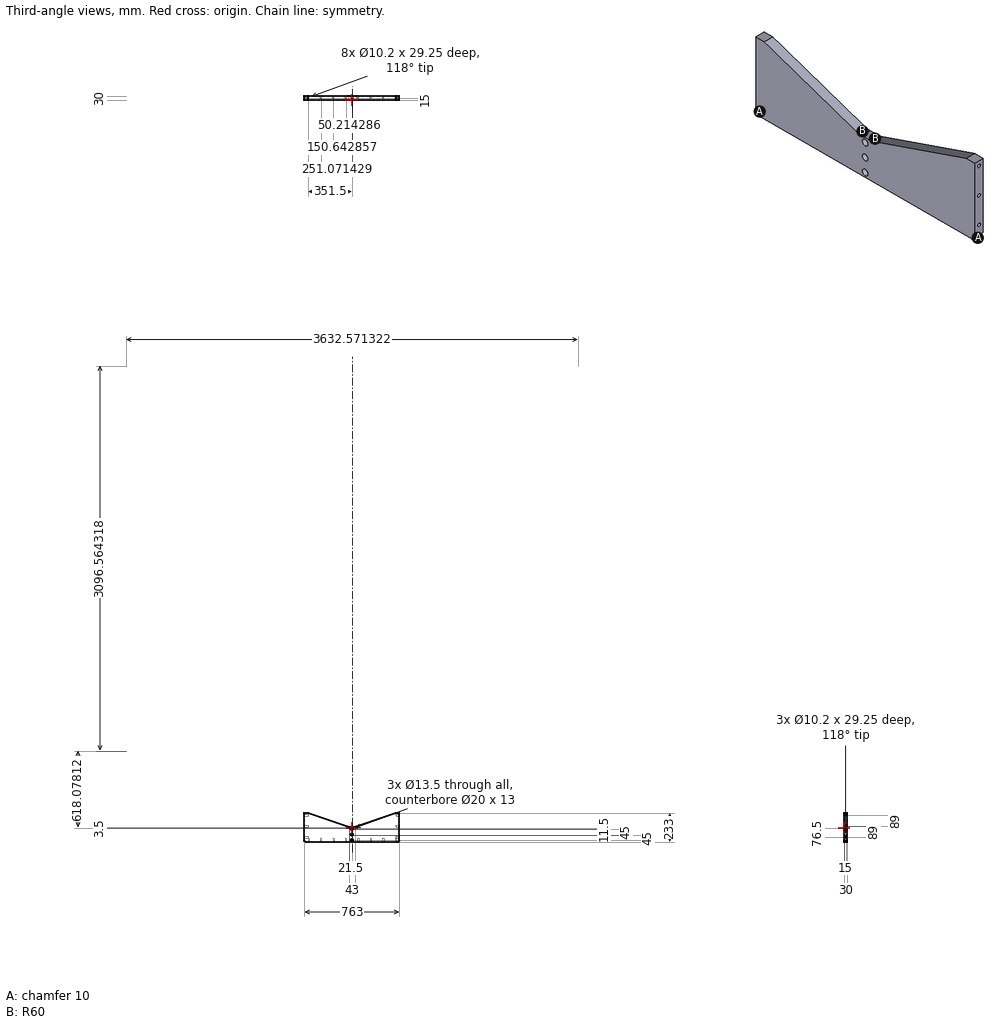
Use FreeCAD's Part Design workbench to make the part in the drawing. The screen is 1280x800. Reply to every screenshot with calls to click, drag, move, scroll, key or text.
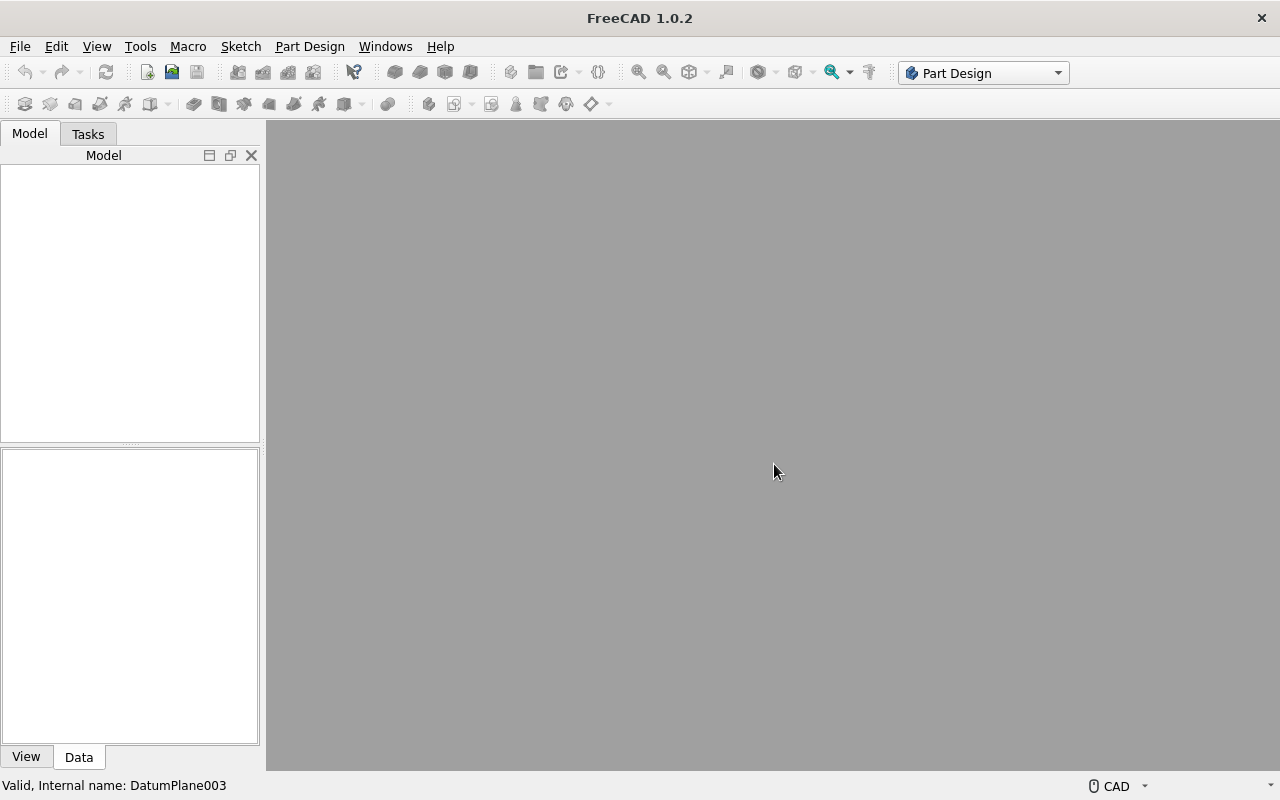
key(ctrl+n)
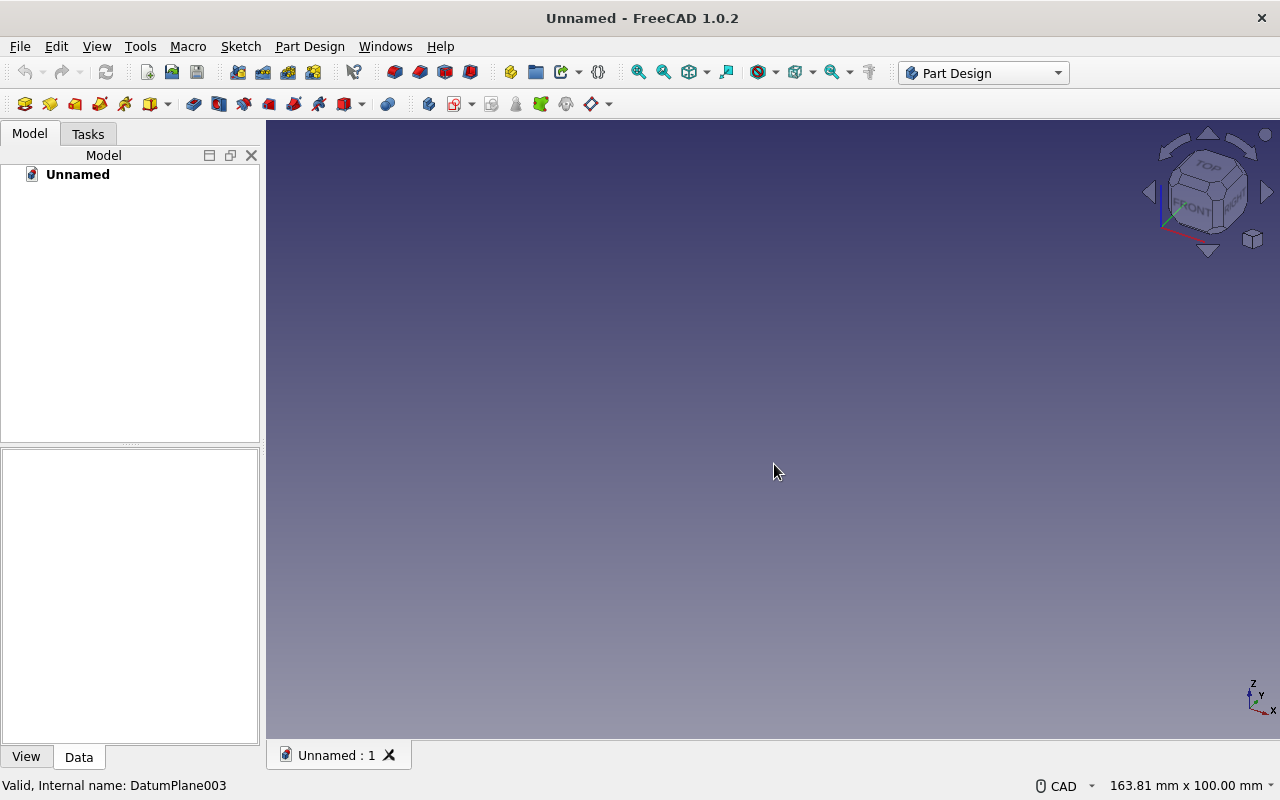
click(454, 104)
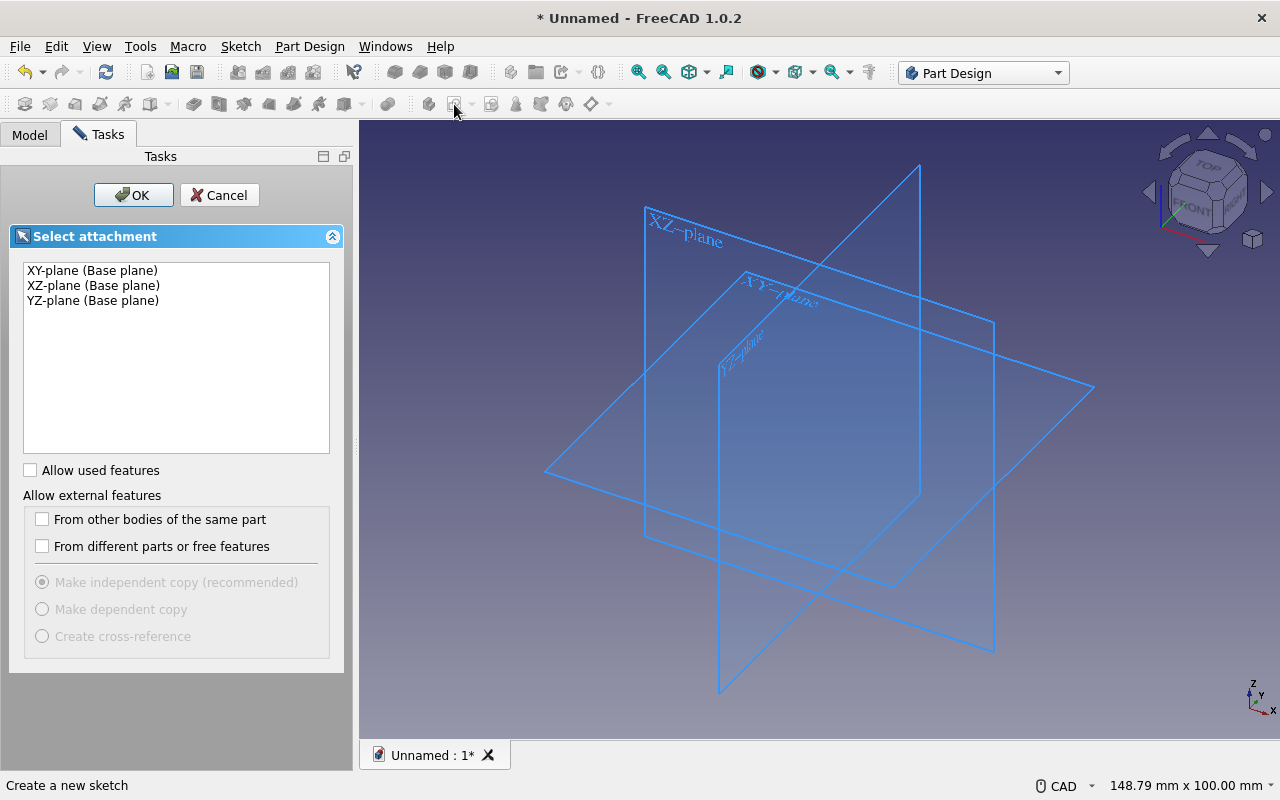
click(84, 286)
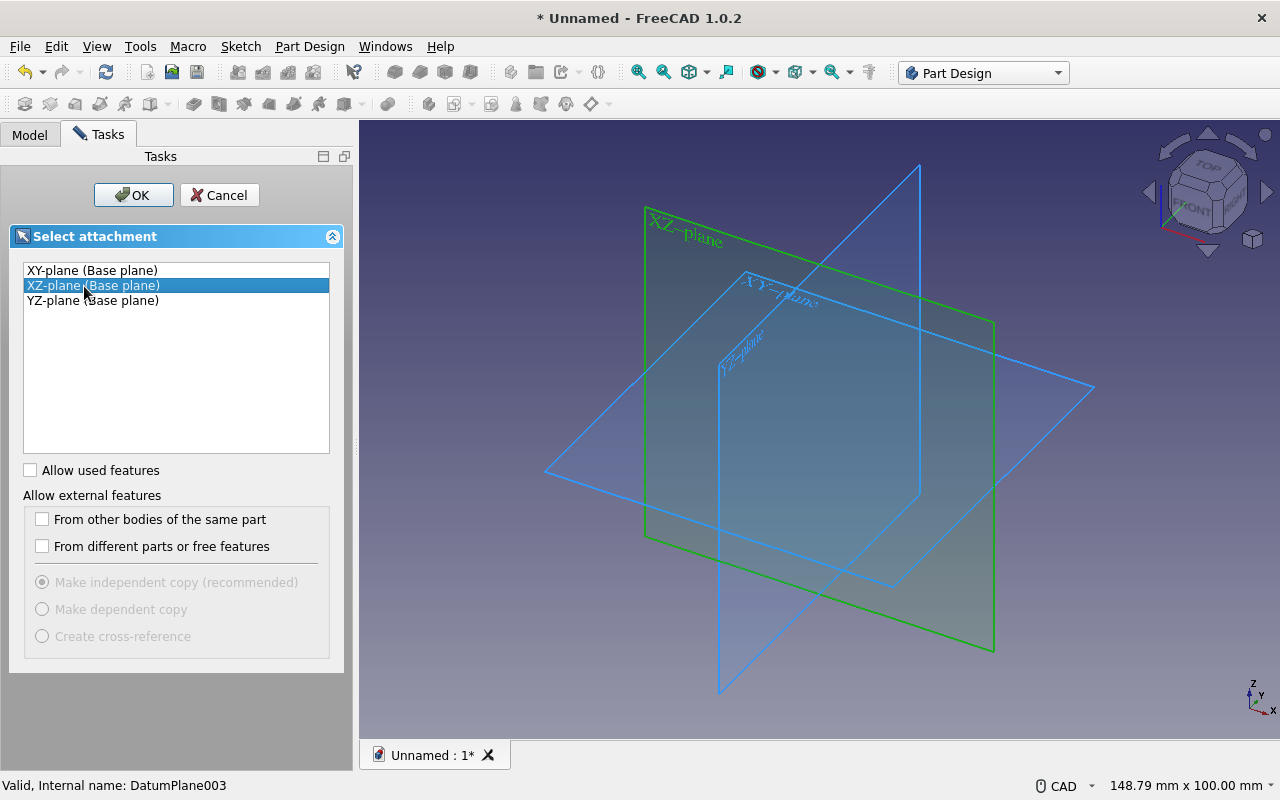
click(134, 195)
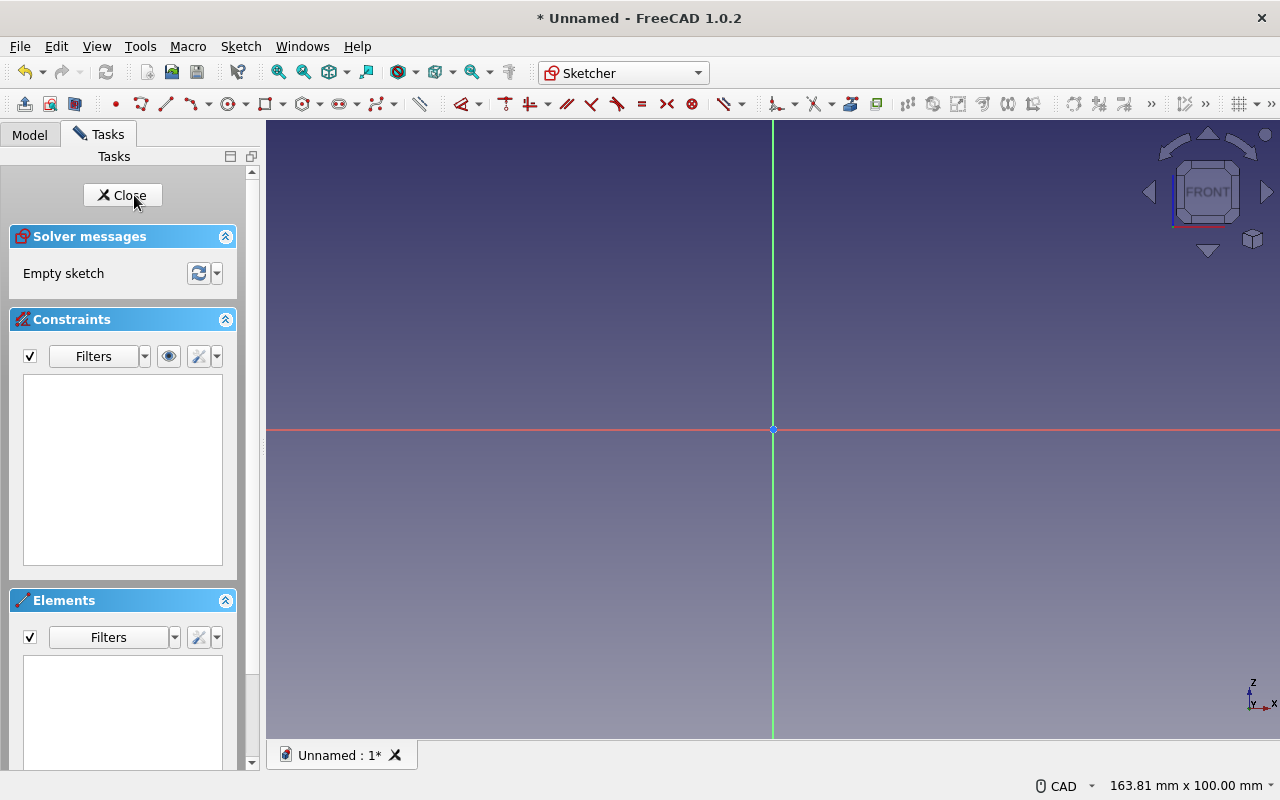
scroll(694, 430, down, 10)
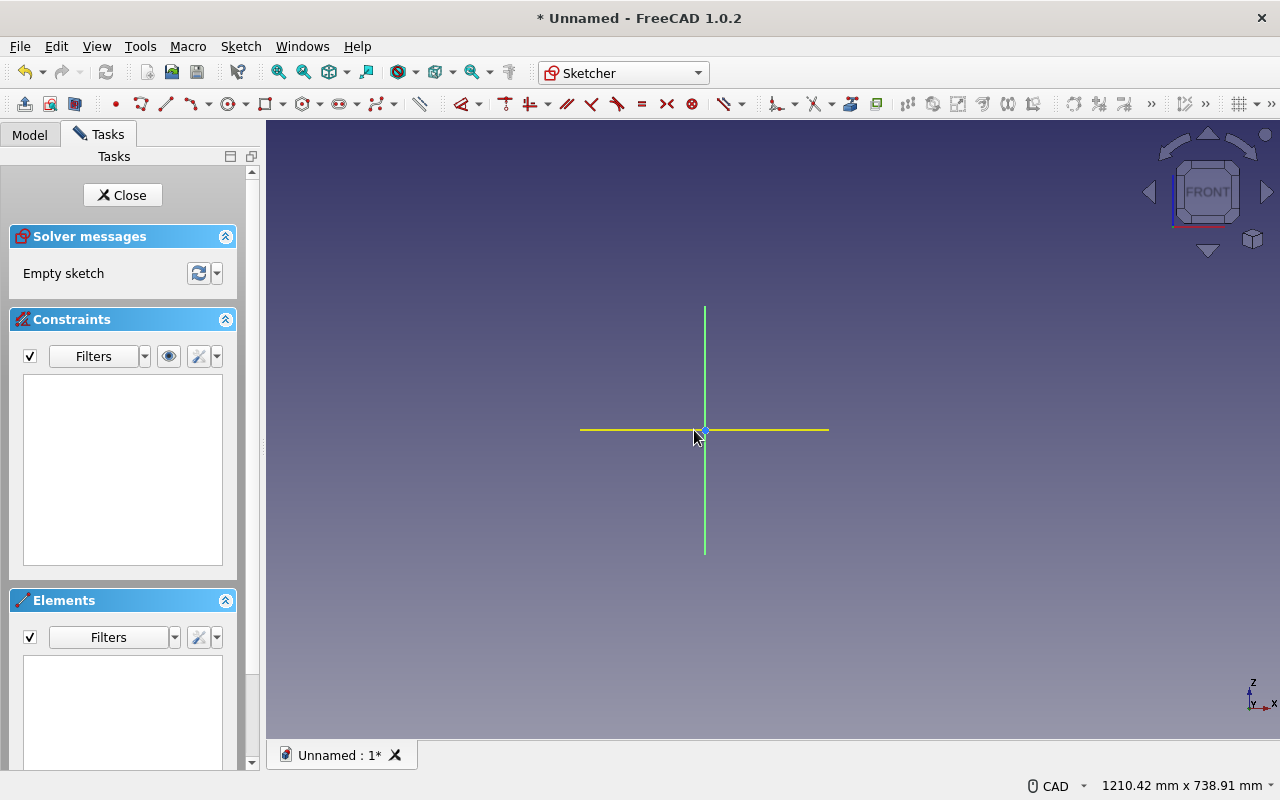
key(g)
key(v)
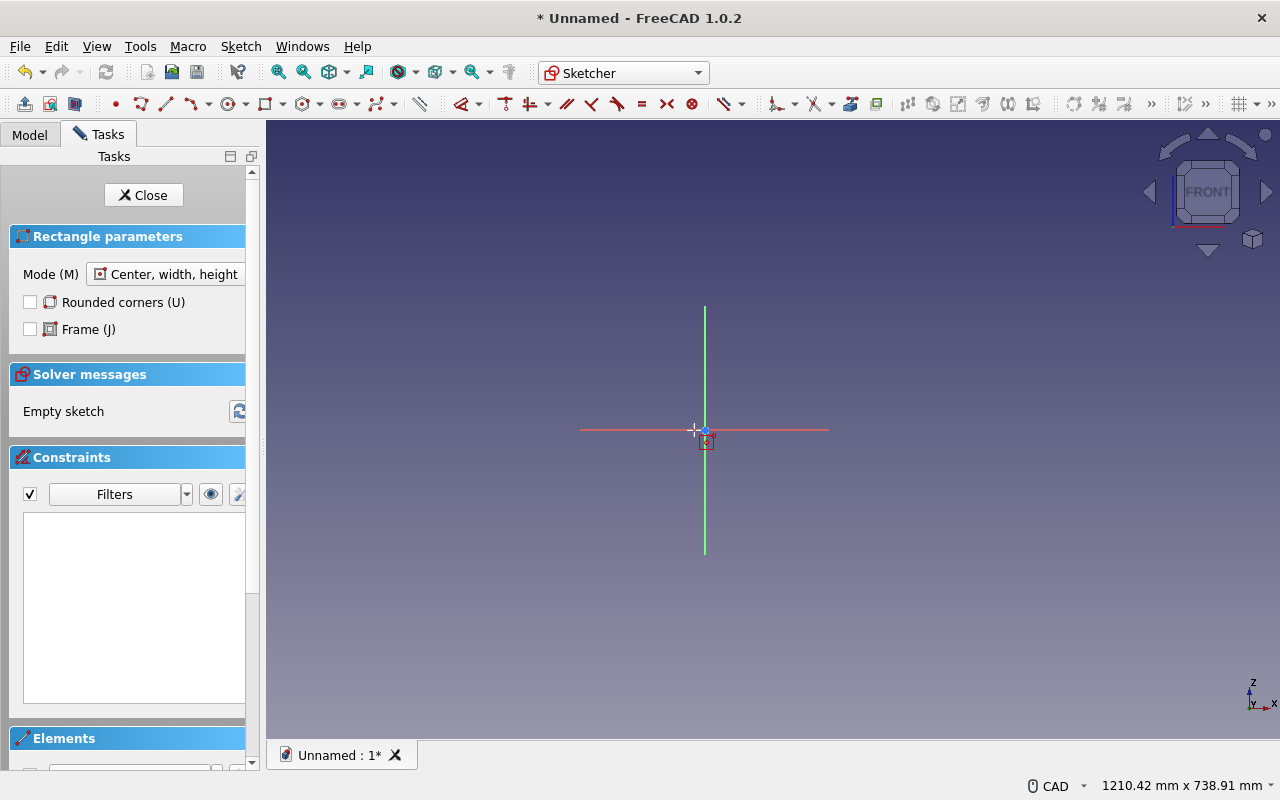
click(705, 430)
click(1025, 333)
key(Escape)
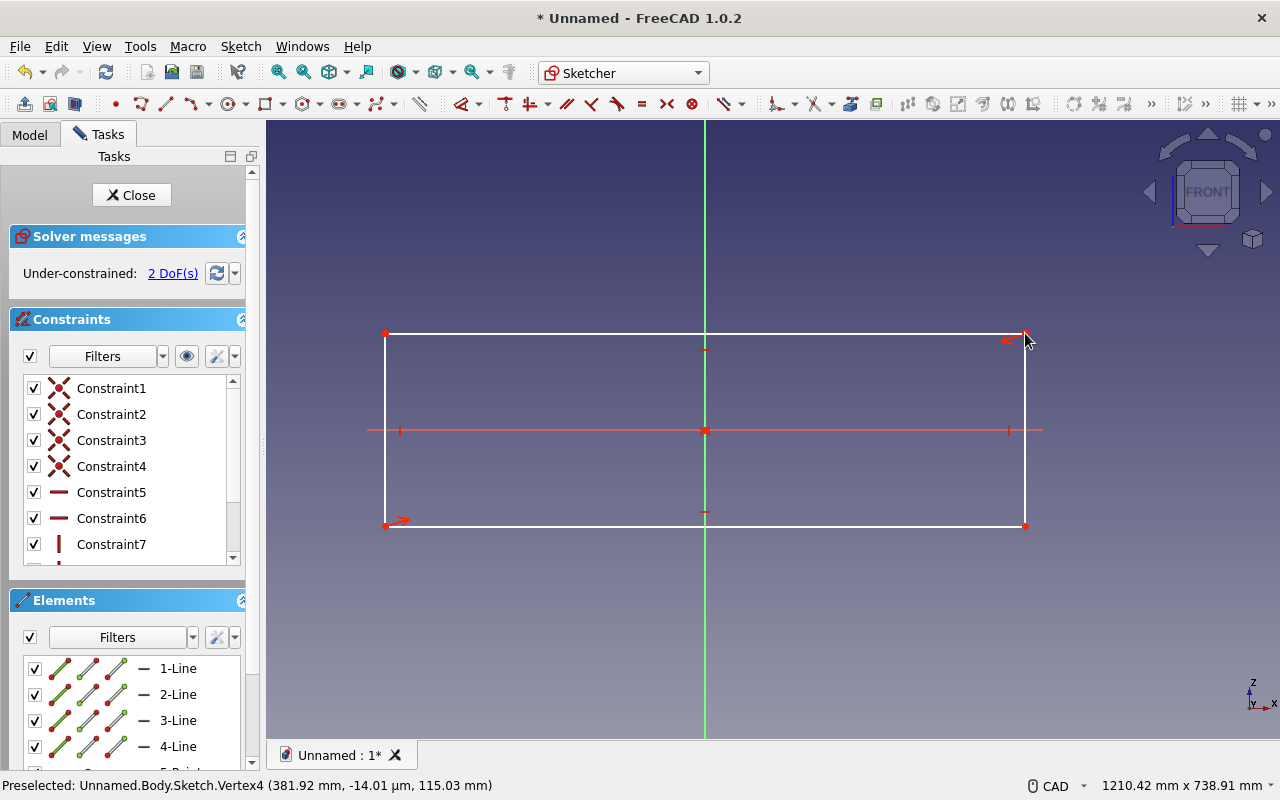
key(d)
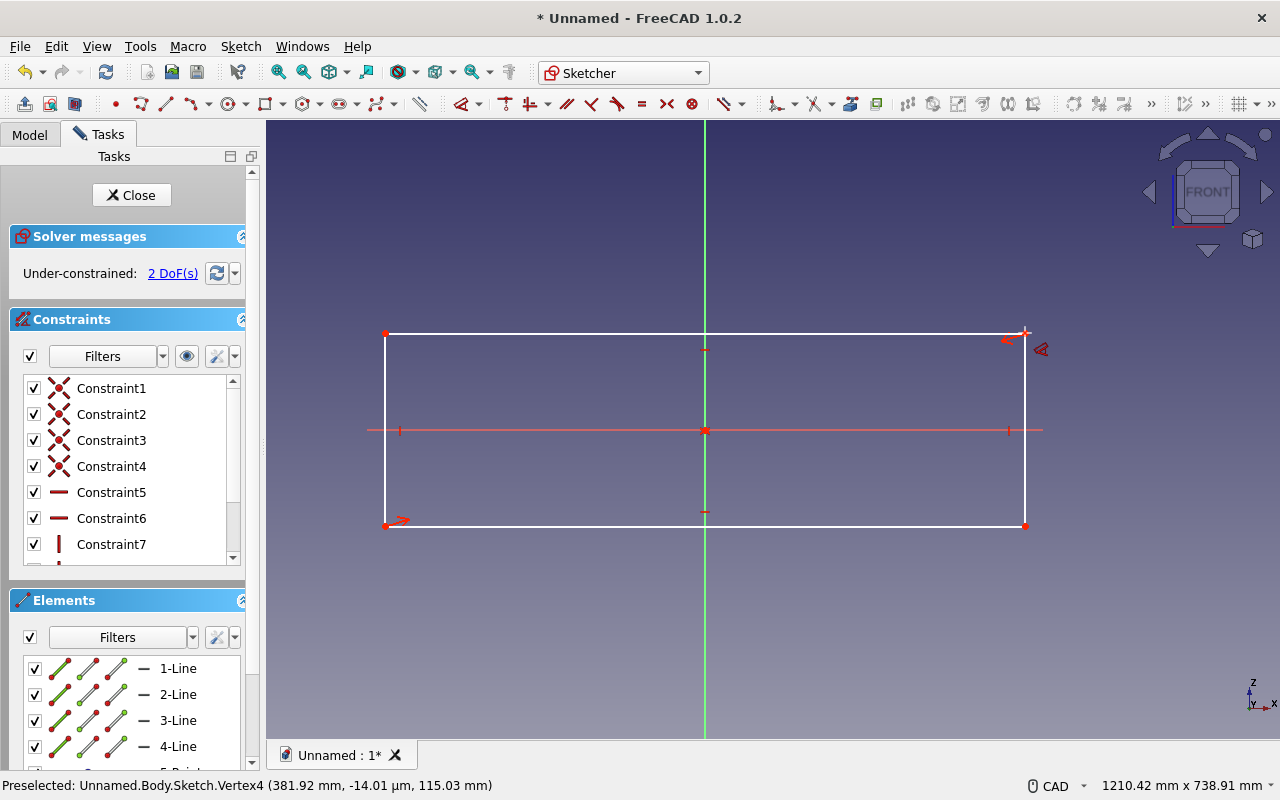
click(577, 527)
click(558, 561)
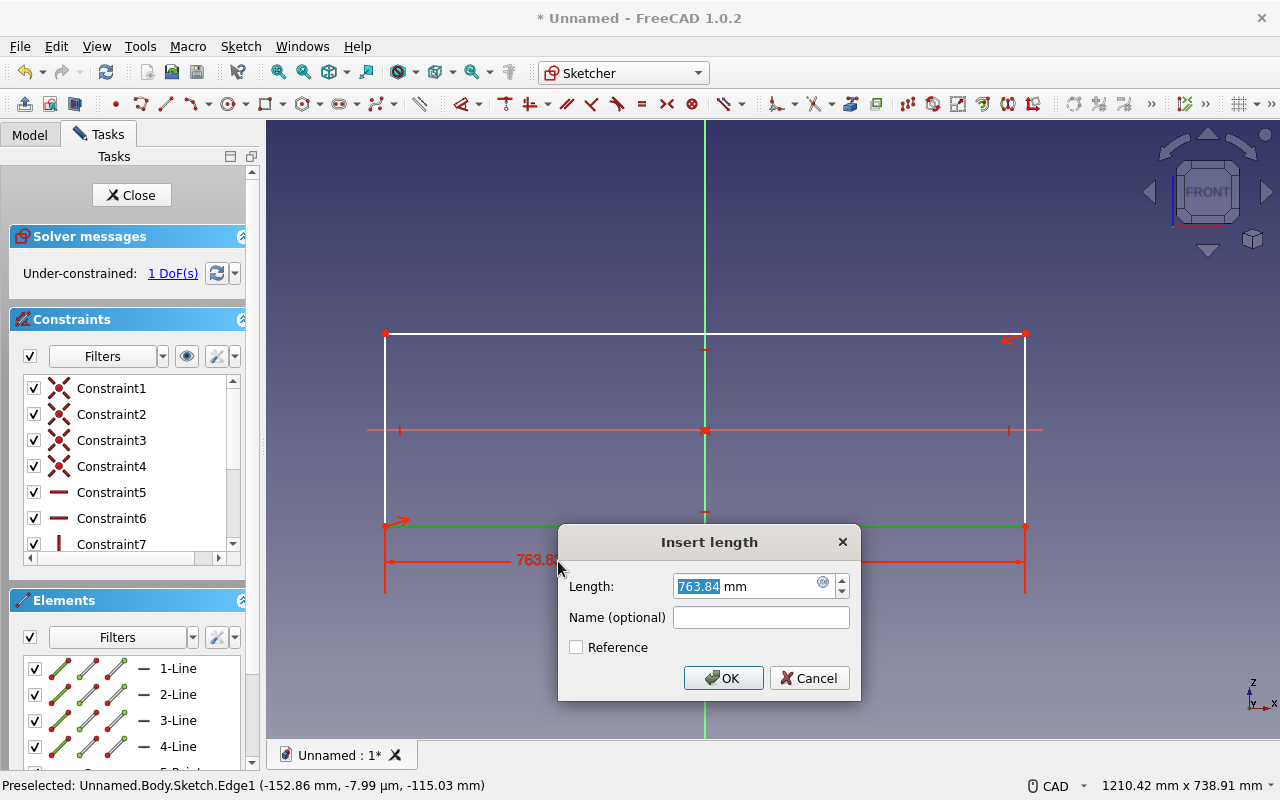
text(763)
key(Return)